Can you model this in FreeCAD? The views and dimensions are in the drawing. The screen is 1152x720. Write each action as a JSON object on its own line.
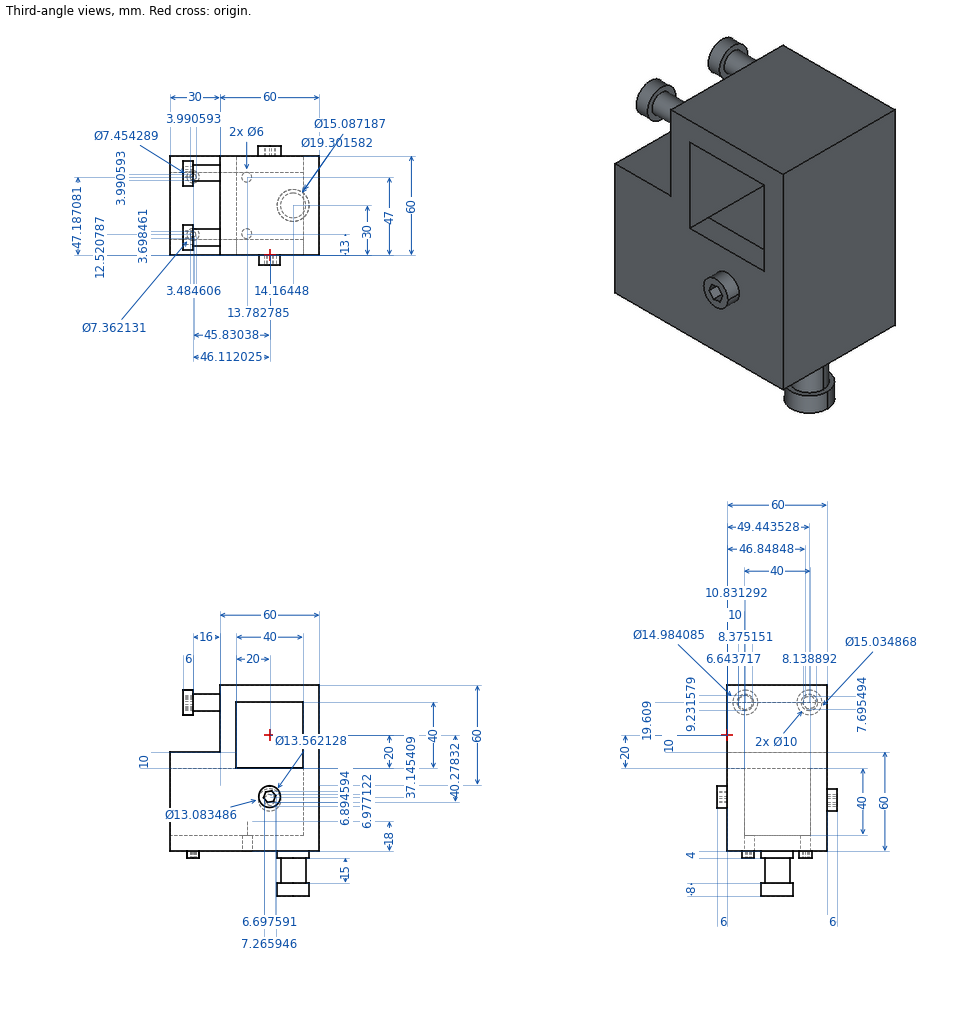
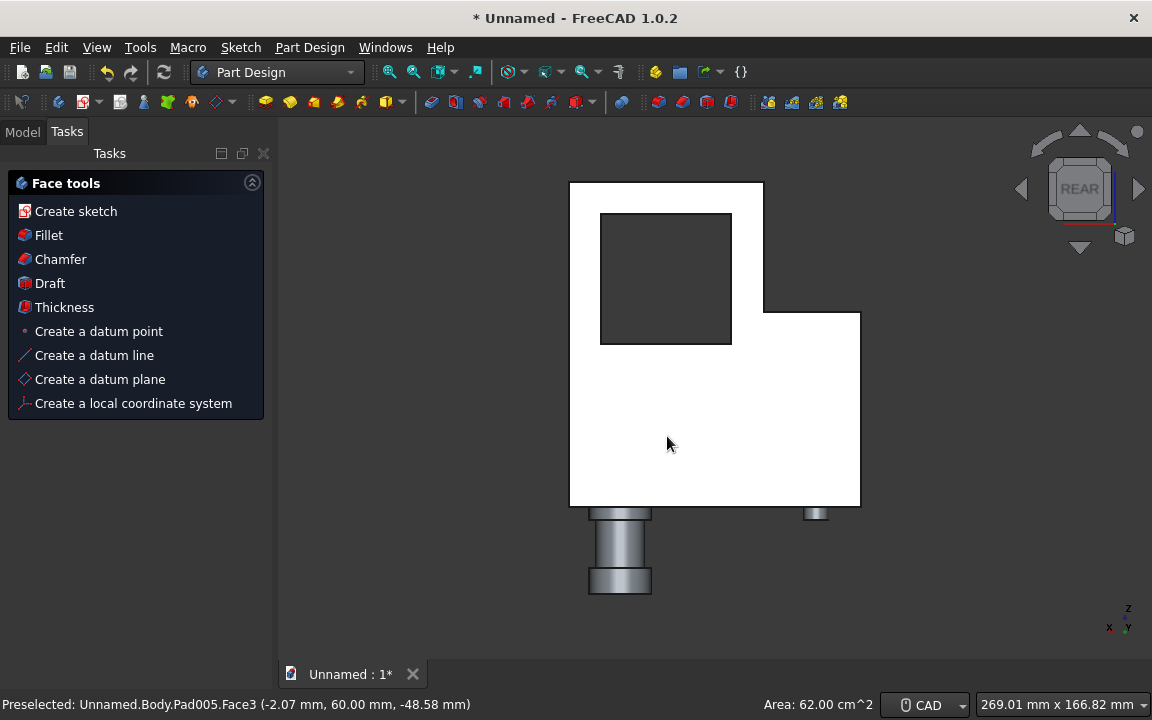
{"action": "left_click", "coordinate": [84, 102]}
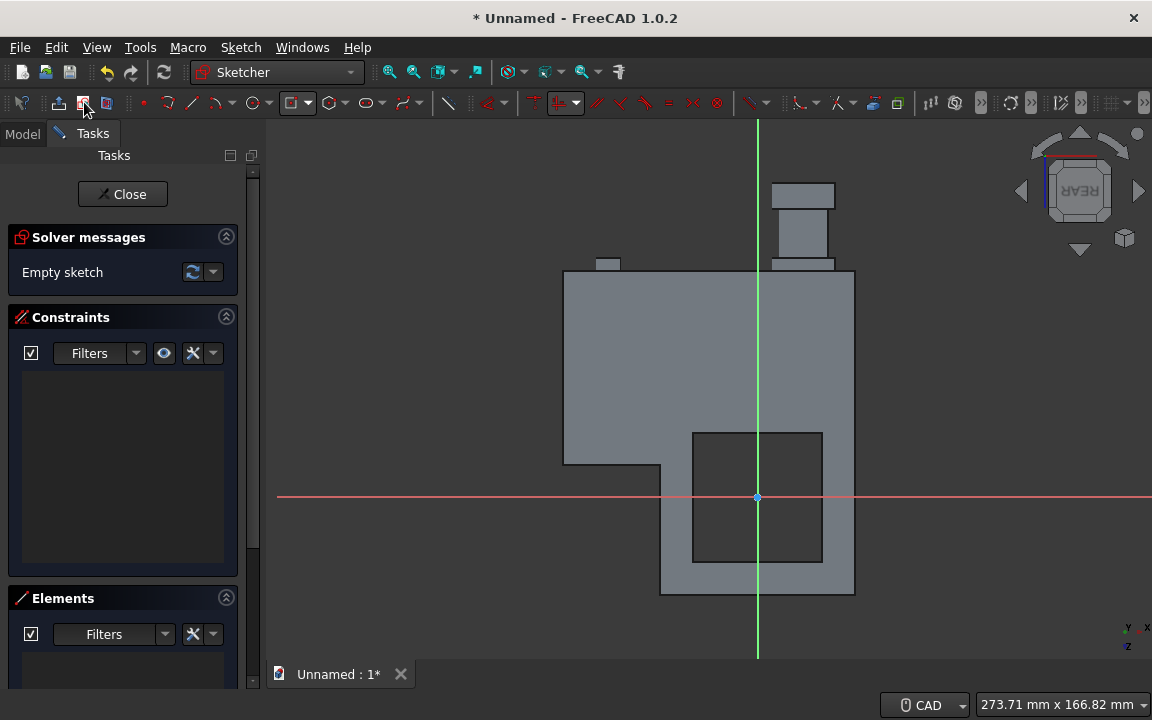
{"action": "scroll", "coordinate": [776, 368], "scroll_direction": "up", "scroll_amount": 10}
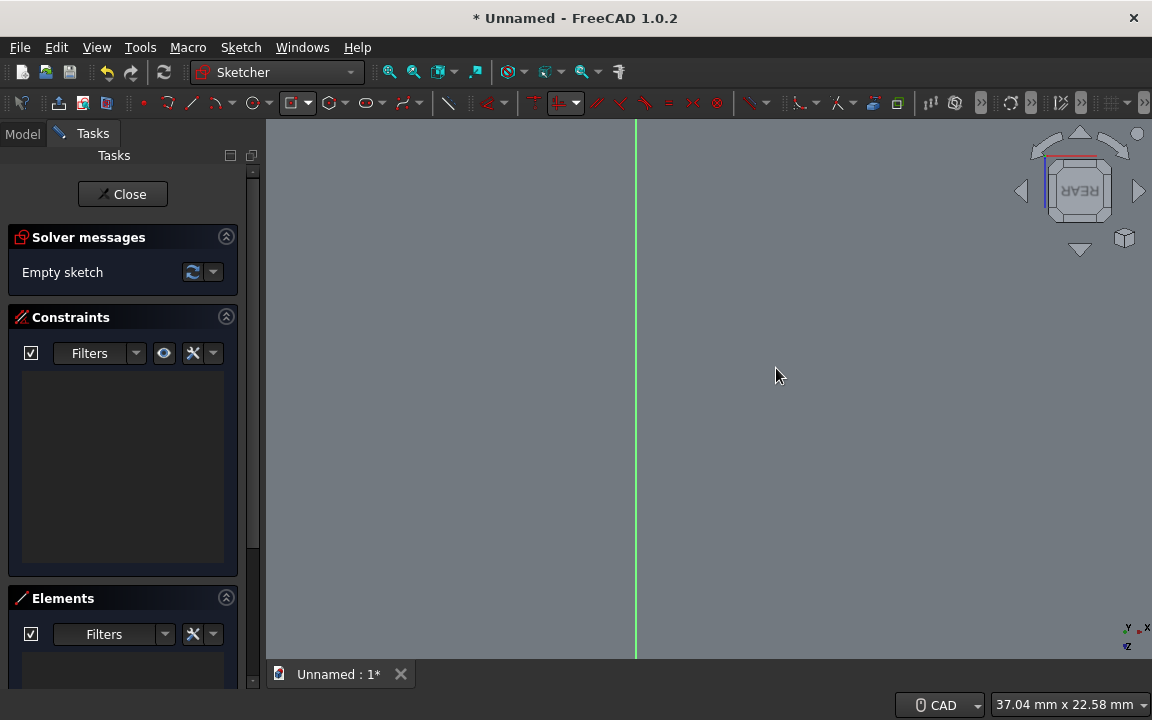
{"action": "left_click", "coordinate": [330, 104]}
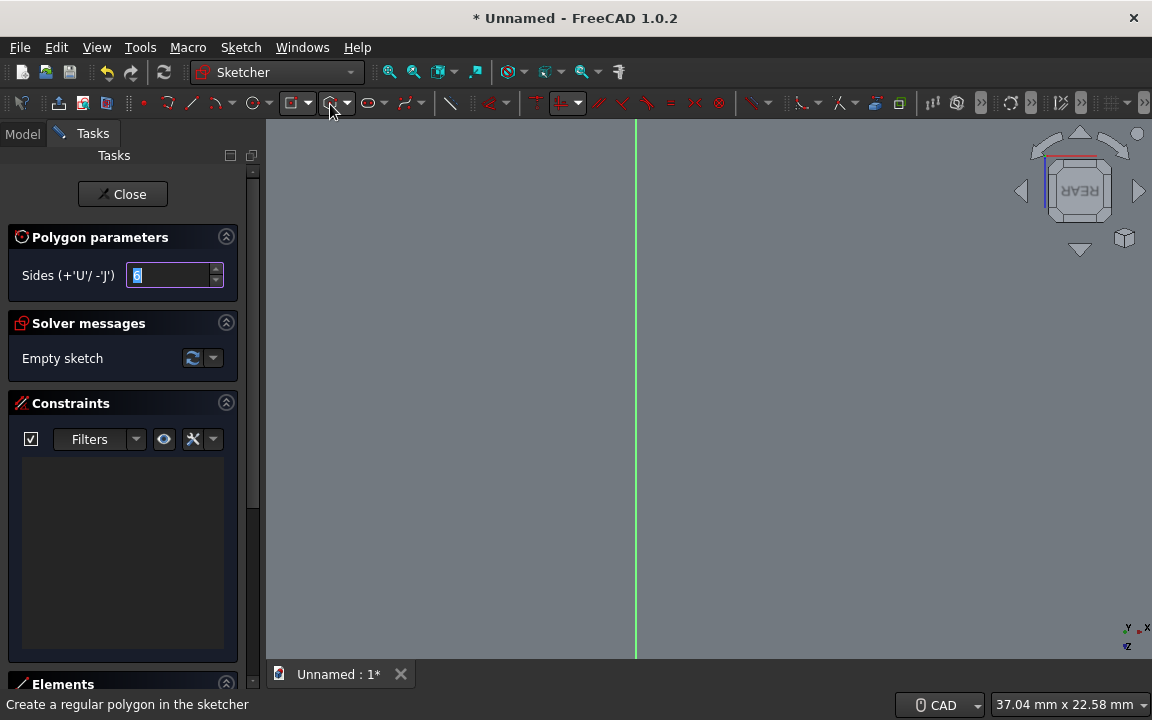
{"action": "left_click", "coordinate": [636, 386]}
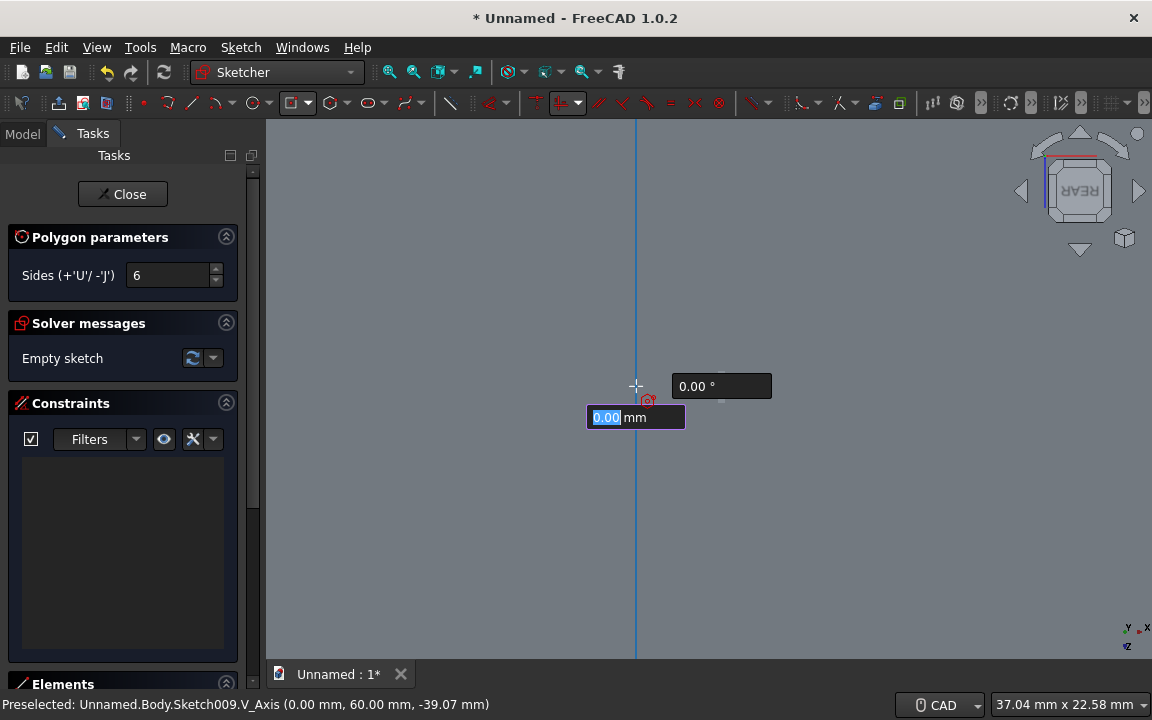
{"action": "left_click", "coordinate": [716, 358]}
{"action": "right_click", "coordinate": [716, 358]}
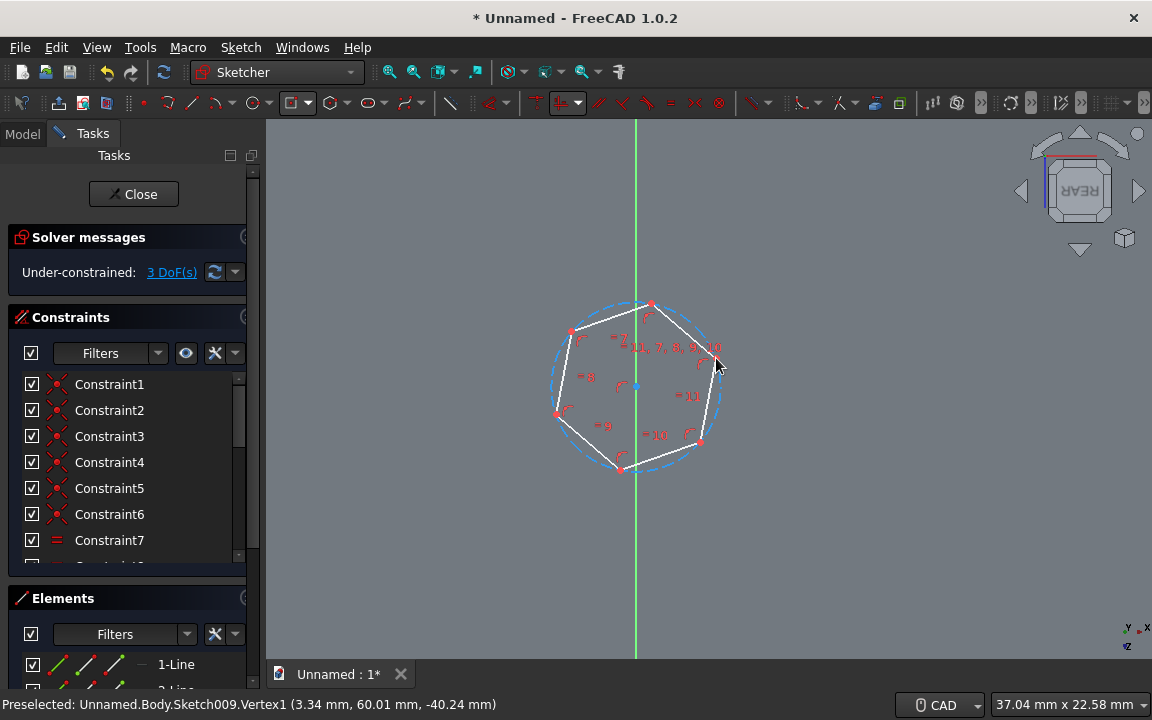
{"action": "left_click", "coordinate": [254, 104]}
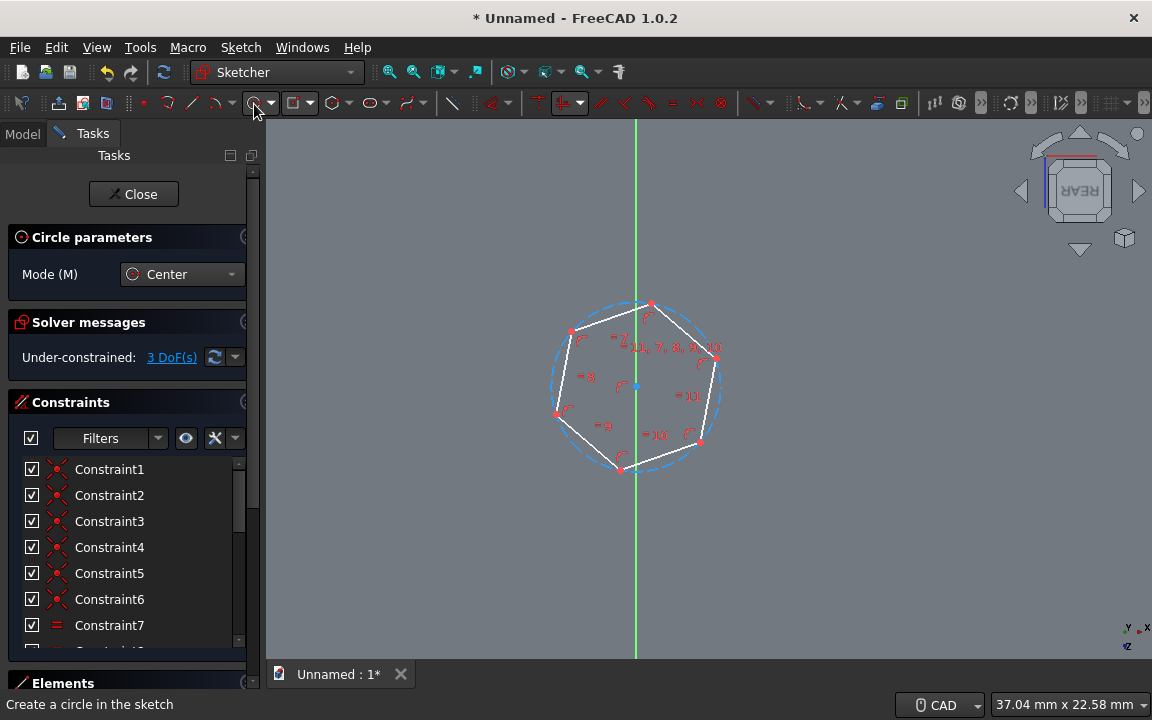
{"action": "left_click", "coordinate": [636, 387]}
{"action": "left_click", "coordinate": [751, 272]}
{"action": "key", "text": "Escape"}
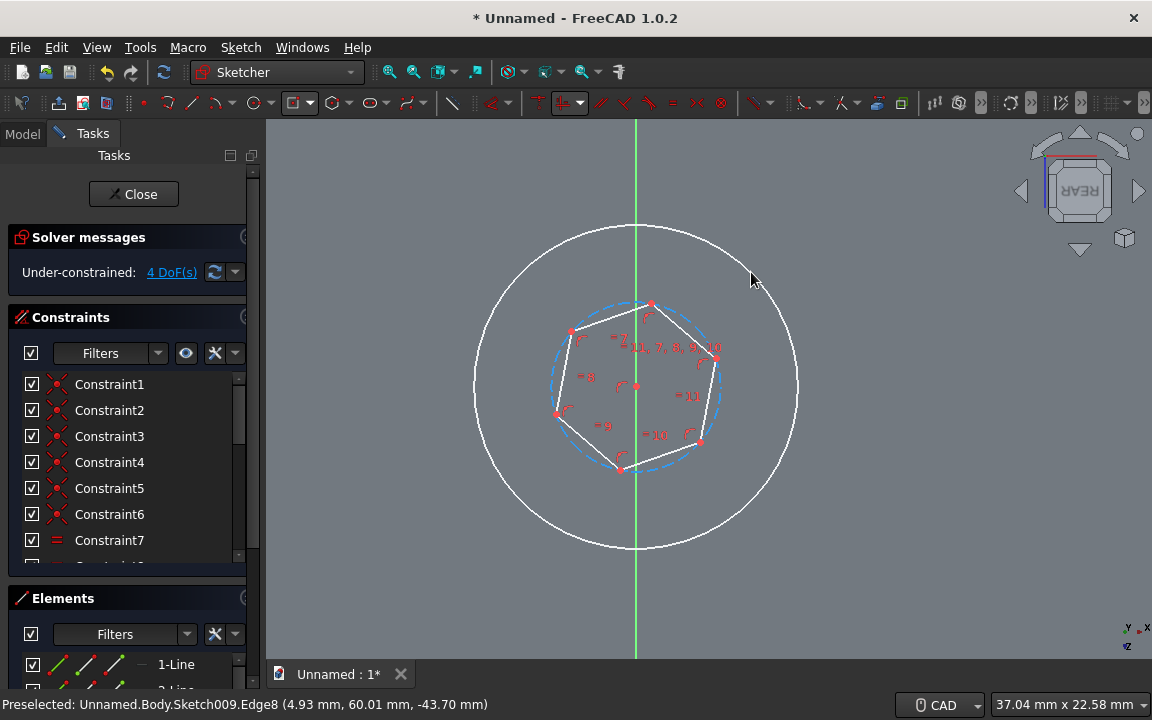
{"action": "left_click", "coordinate": [492, 104]}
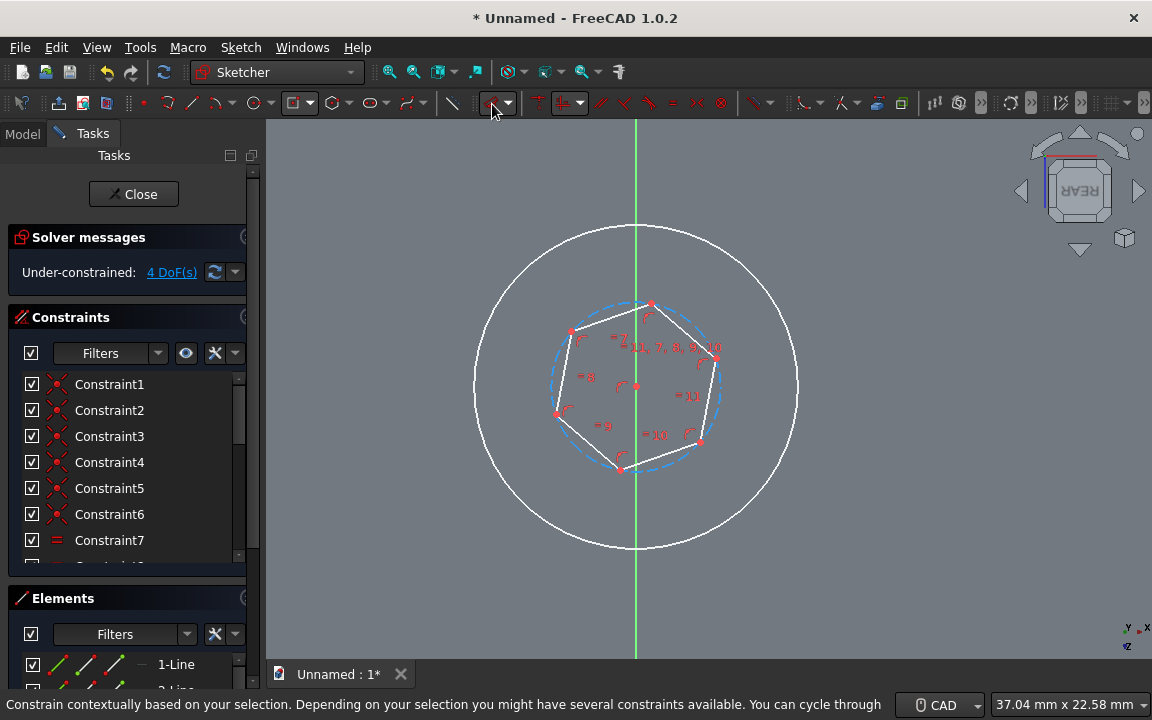
{"action": "left_click", "coordinate": [750, 272]}
{"action": "left_click", "coordinate": [773, 249]}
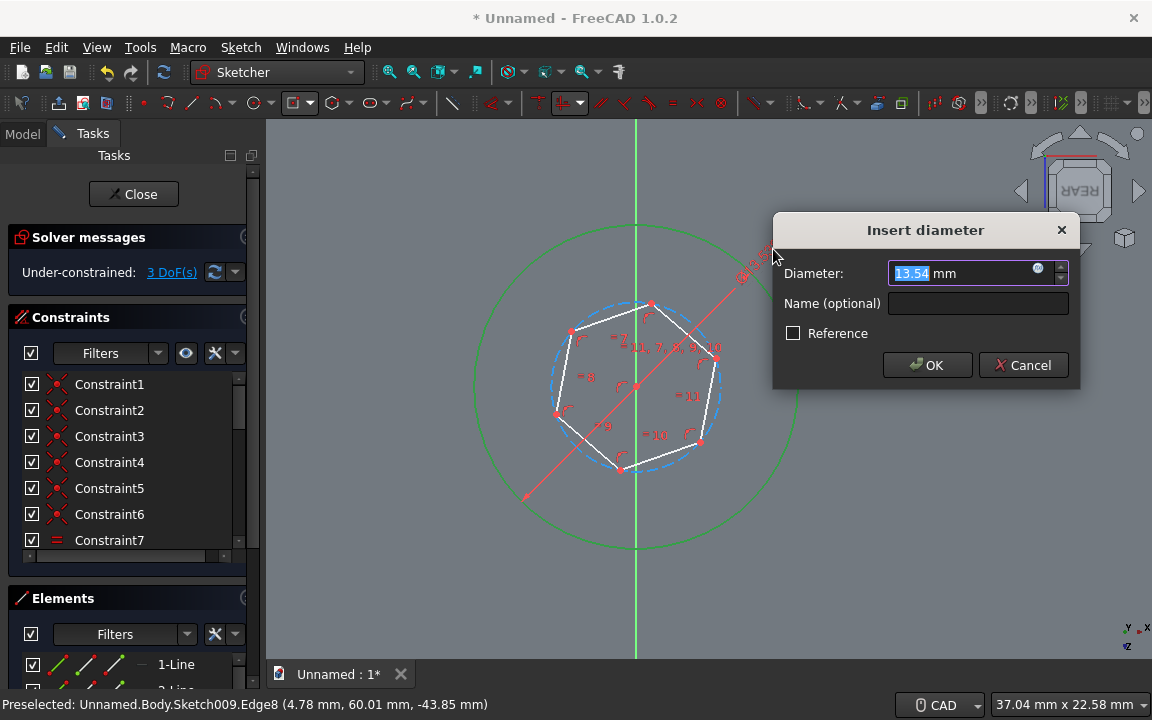
{"action": "type", "text": "13.562128"}
{"action": "key", "text": "Return"}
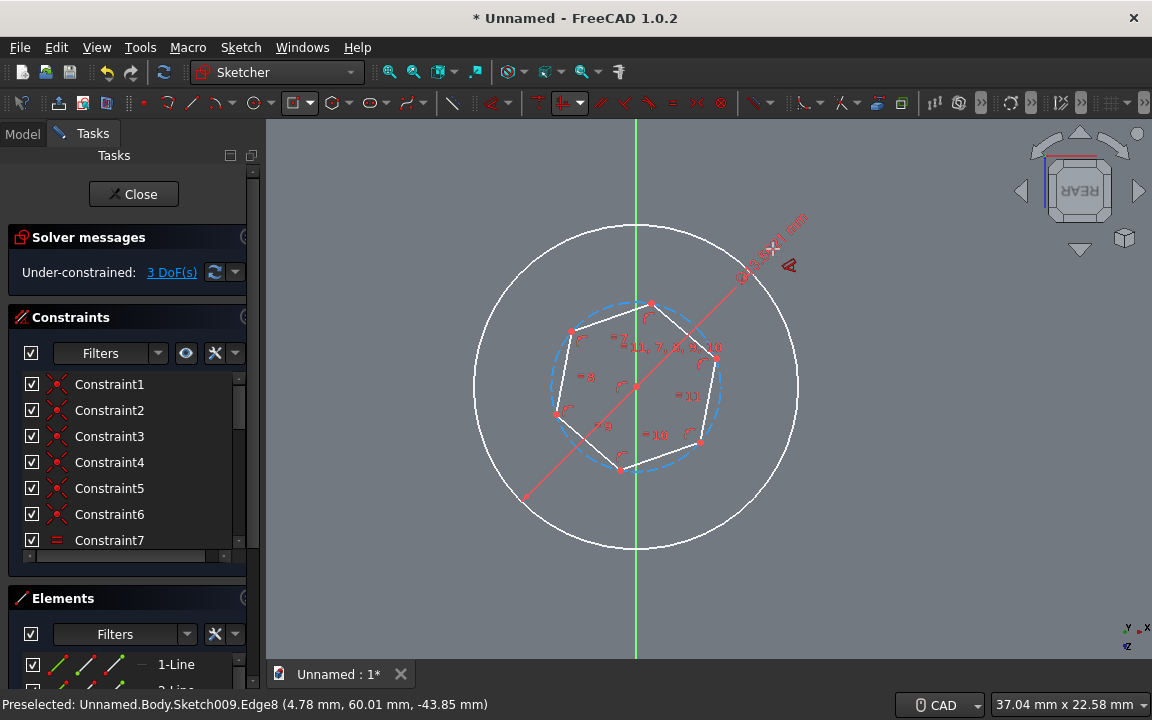
{"action": "left_click", "coordinate": [556, 415]}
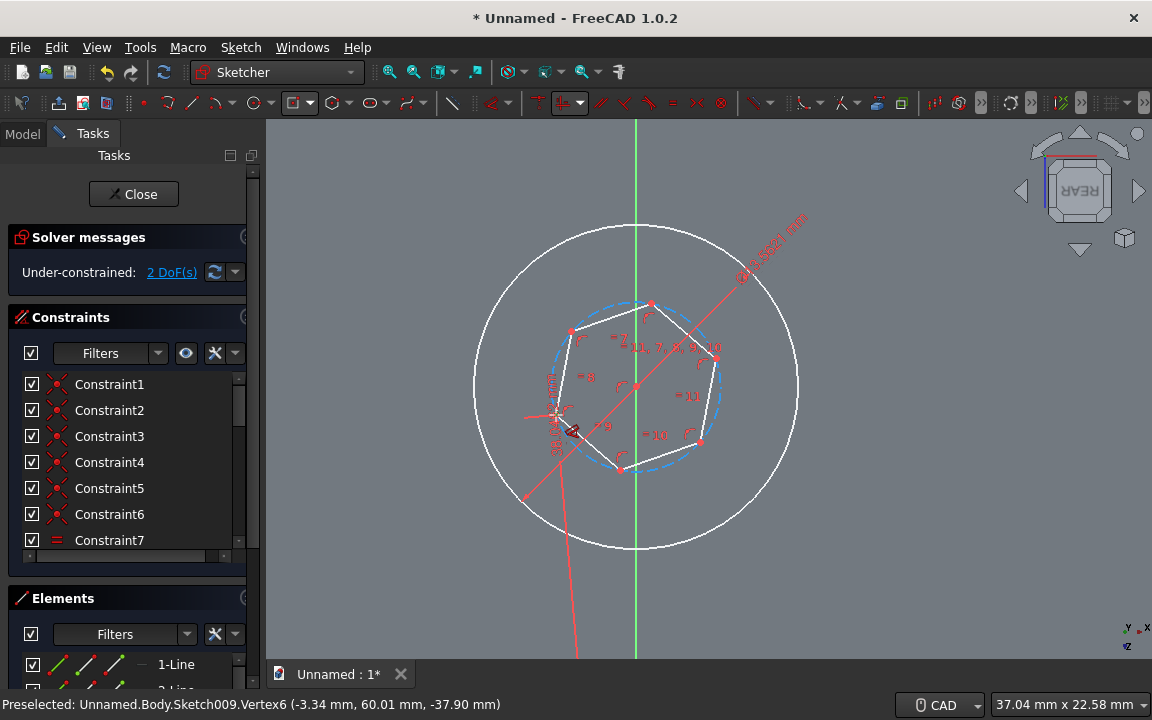
{"action": "left_click", "coordinate": [716, 359]}
{"action": "left_click", "coordinate": [580, 473]}